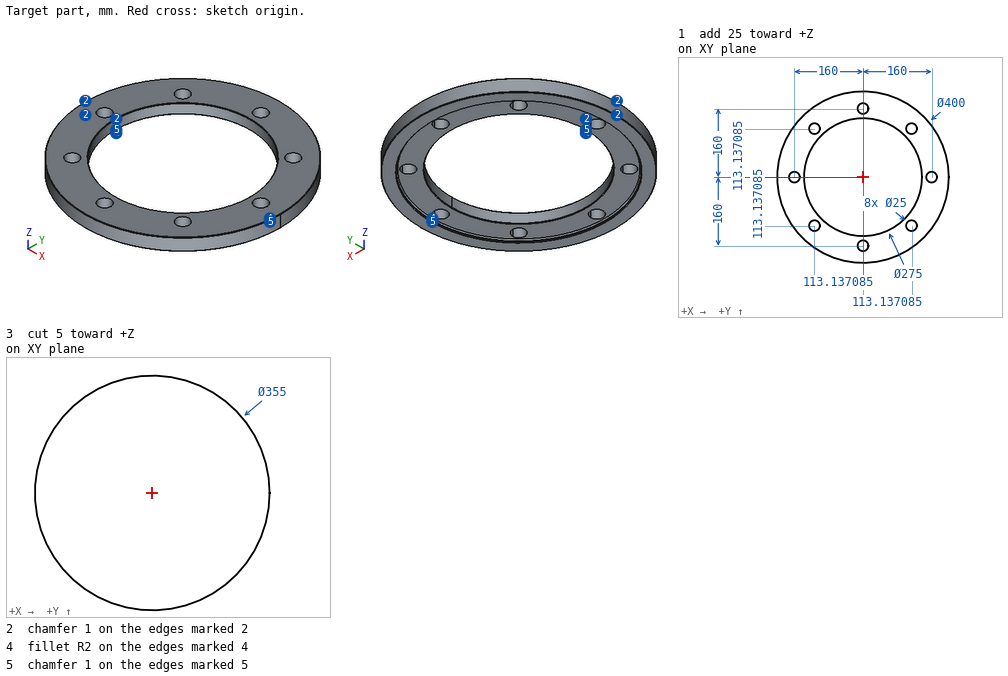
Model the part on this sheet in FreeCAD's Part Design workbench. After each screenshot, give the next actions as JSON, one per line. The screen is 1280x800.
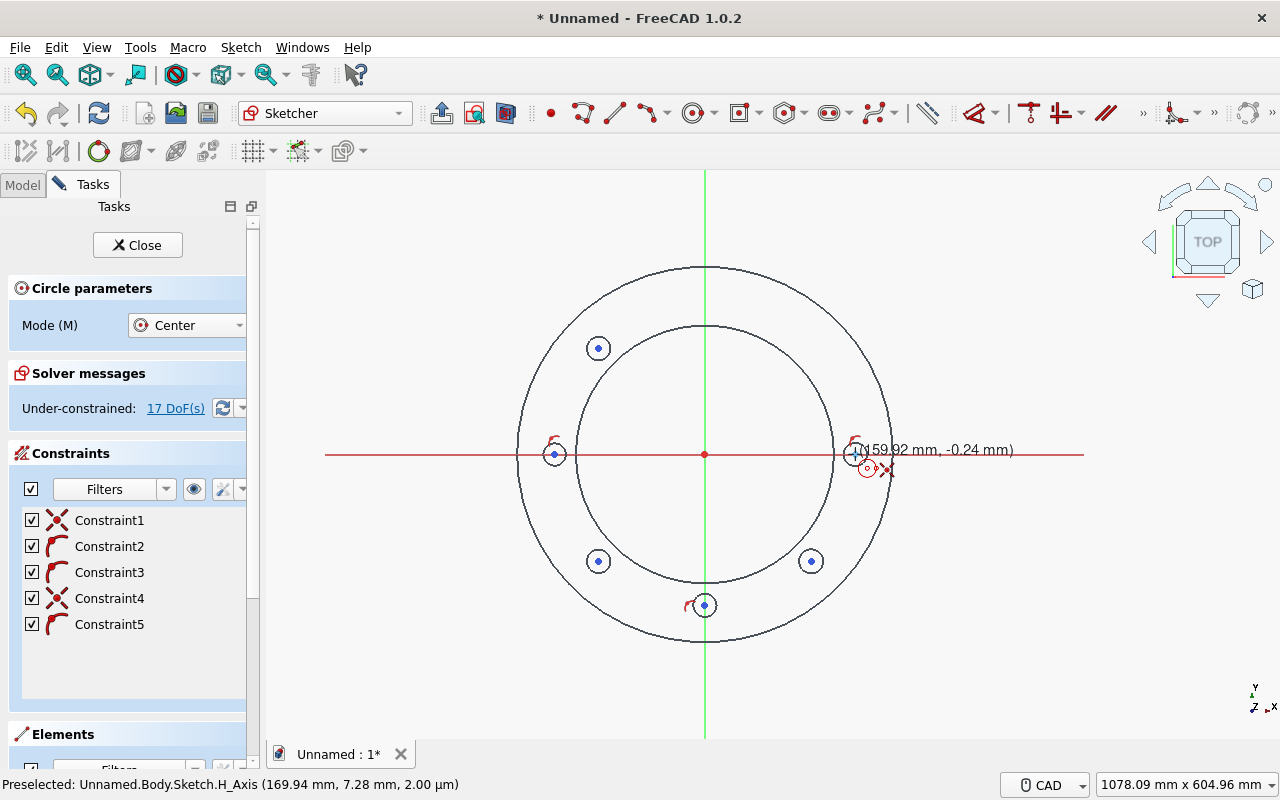
{"action": "scroll", "coordinate": [705, 304], "scroll_direction": "up", "scroll_amount": 4}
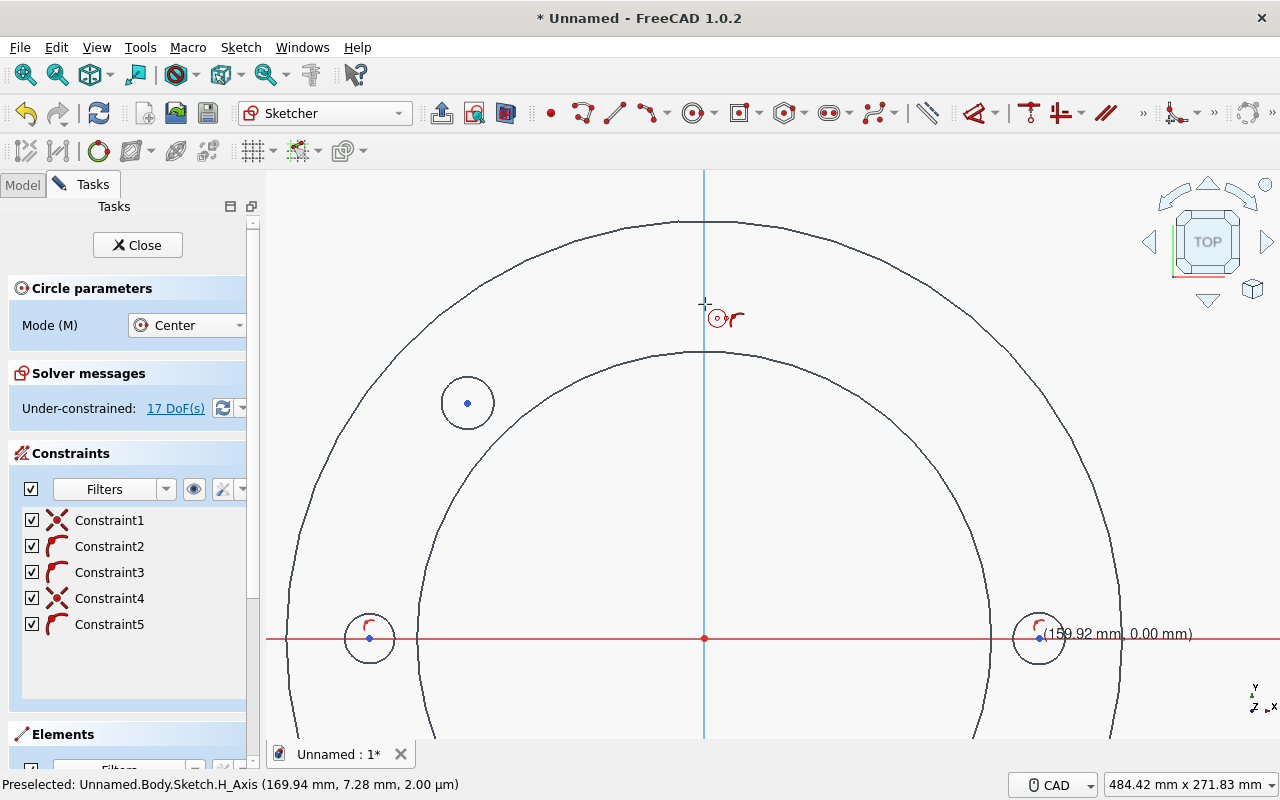
{"action": "left_click", "coordinate": [704, 304]}
{"action": "left_click", "coordinate": [723, 285]}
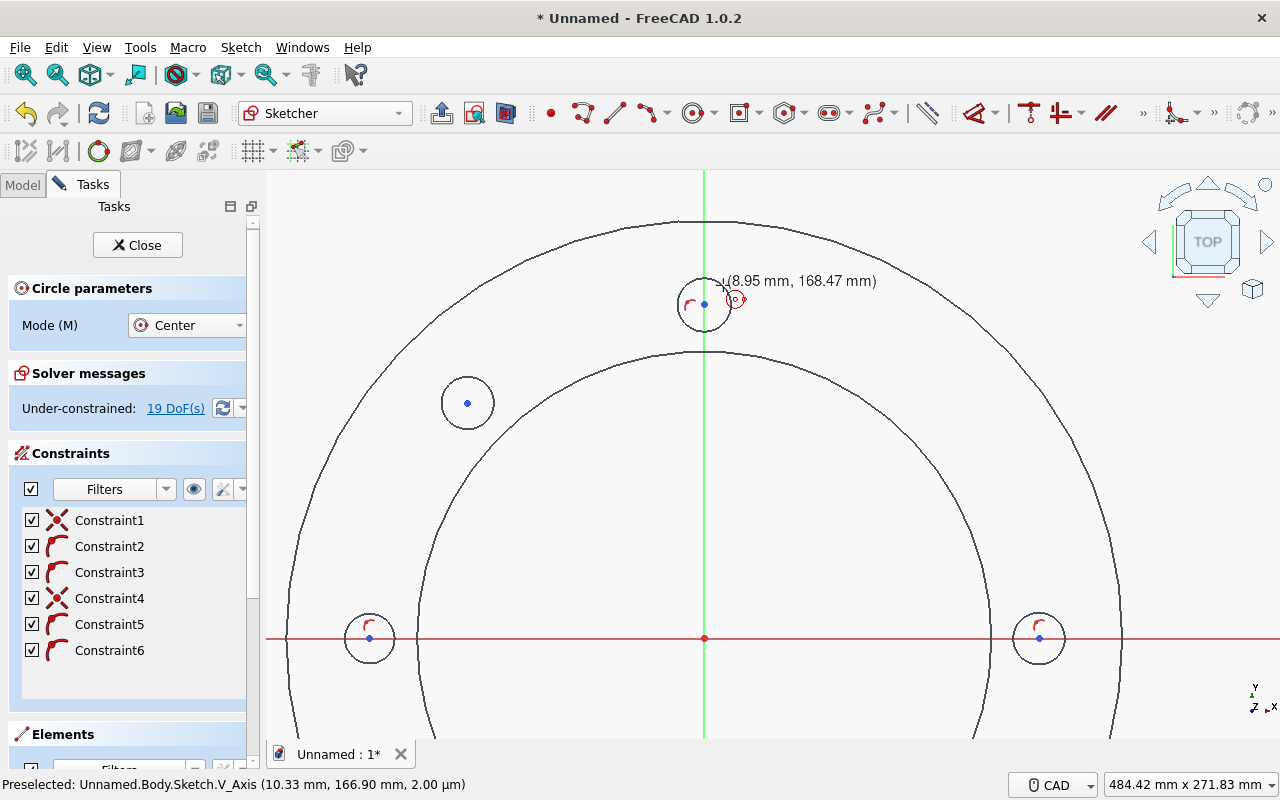
{"action": "left_click", "coordinate": [941, 402]}
{"action": "left_click", "coordinate": [960, 383]}
{"action": "key", "text": "Escape"}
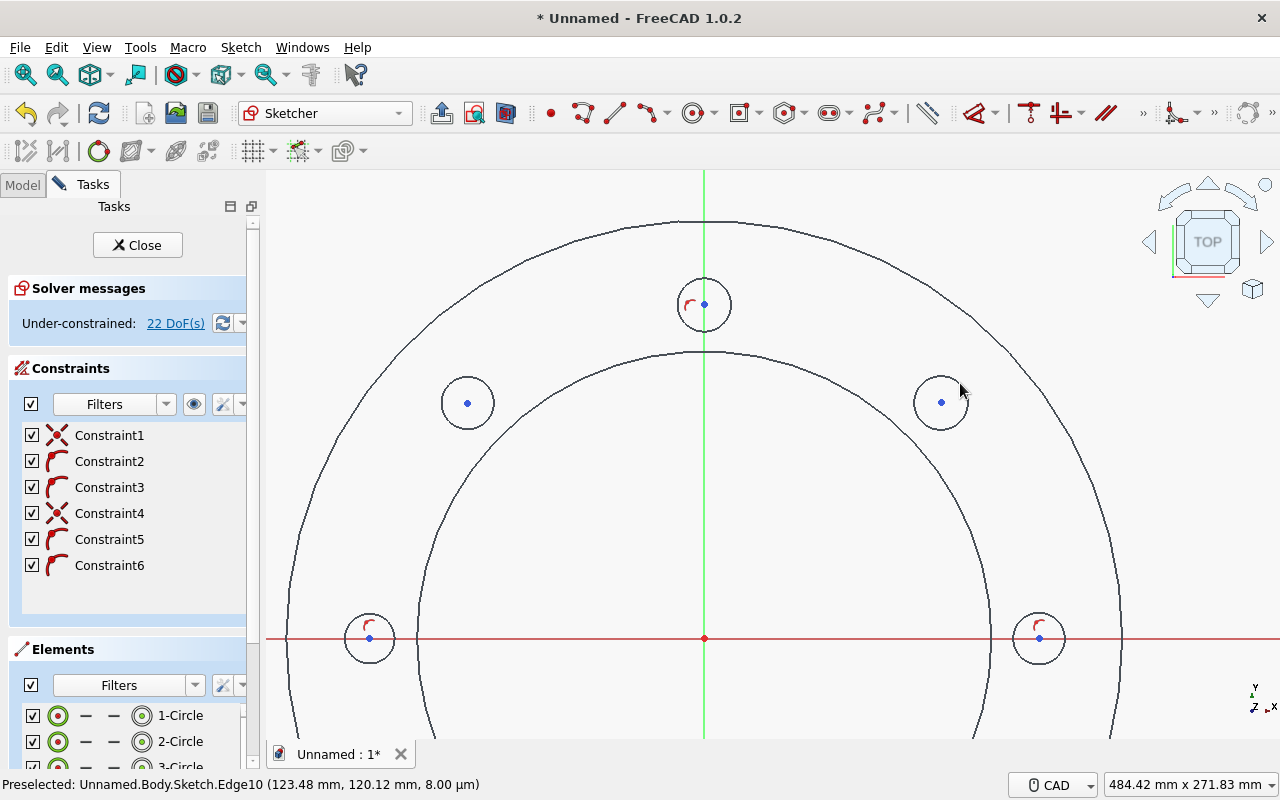
{"action": "scroll", "coordinate": [705, 304], "scroll_direction": "down", "scroll_amount": 4}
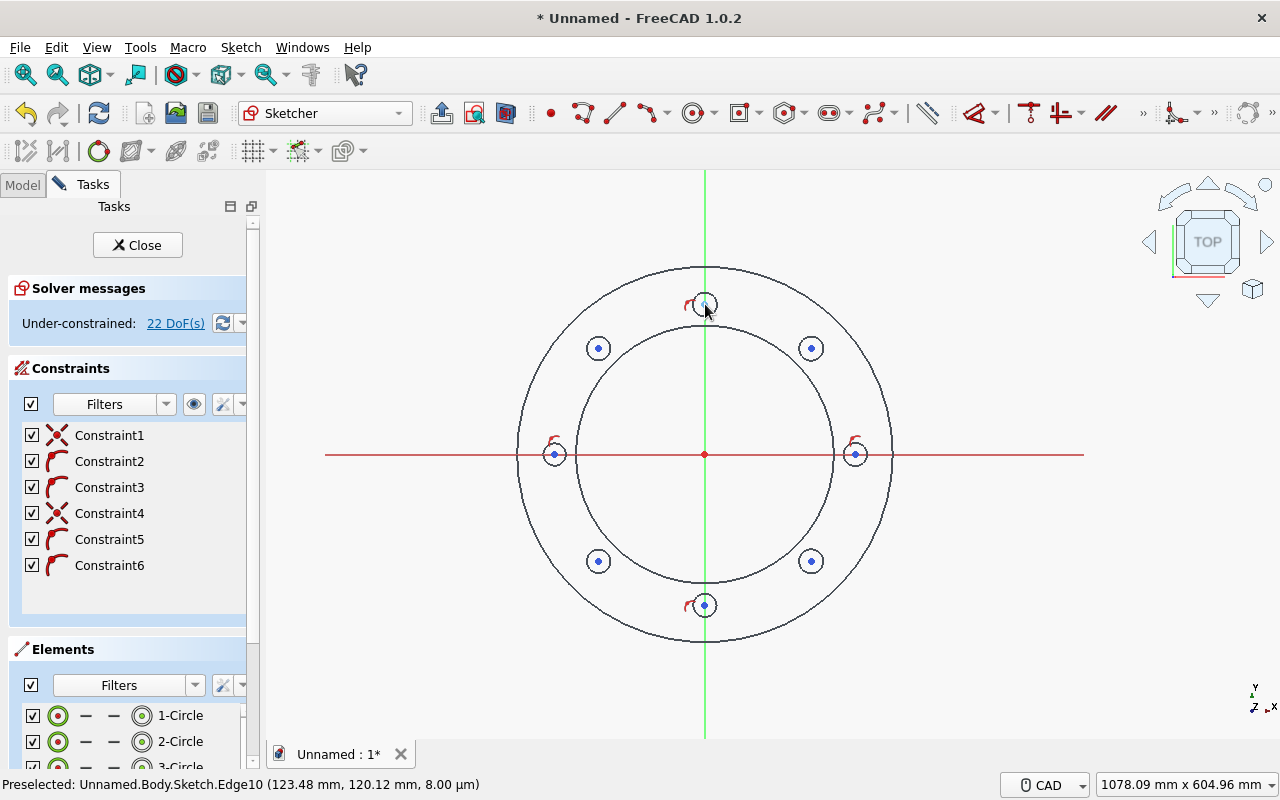
{"action": "scroll", "coordinate": [607, 553], "scroll_direction": "up", "scroll_amount": 2}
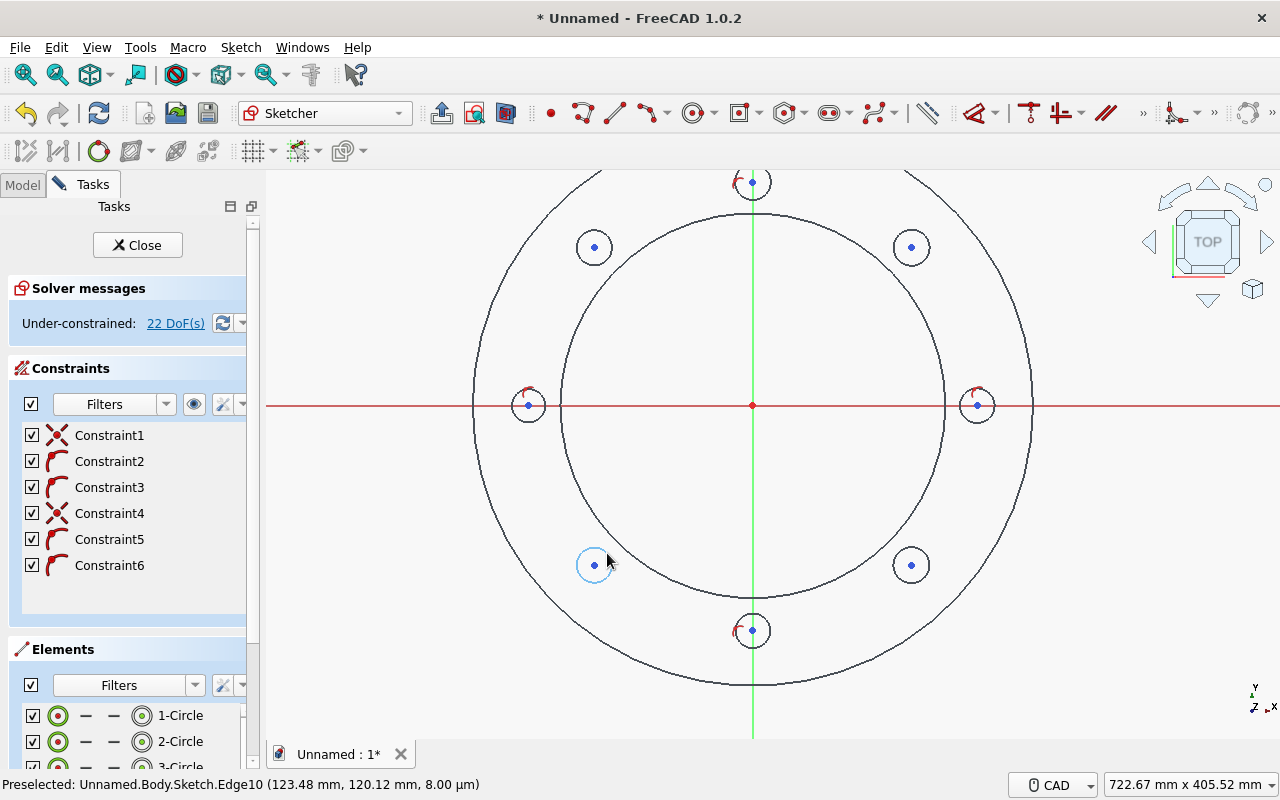
{"action": "left_click", "coordinate": [607, 553]}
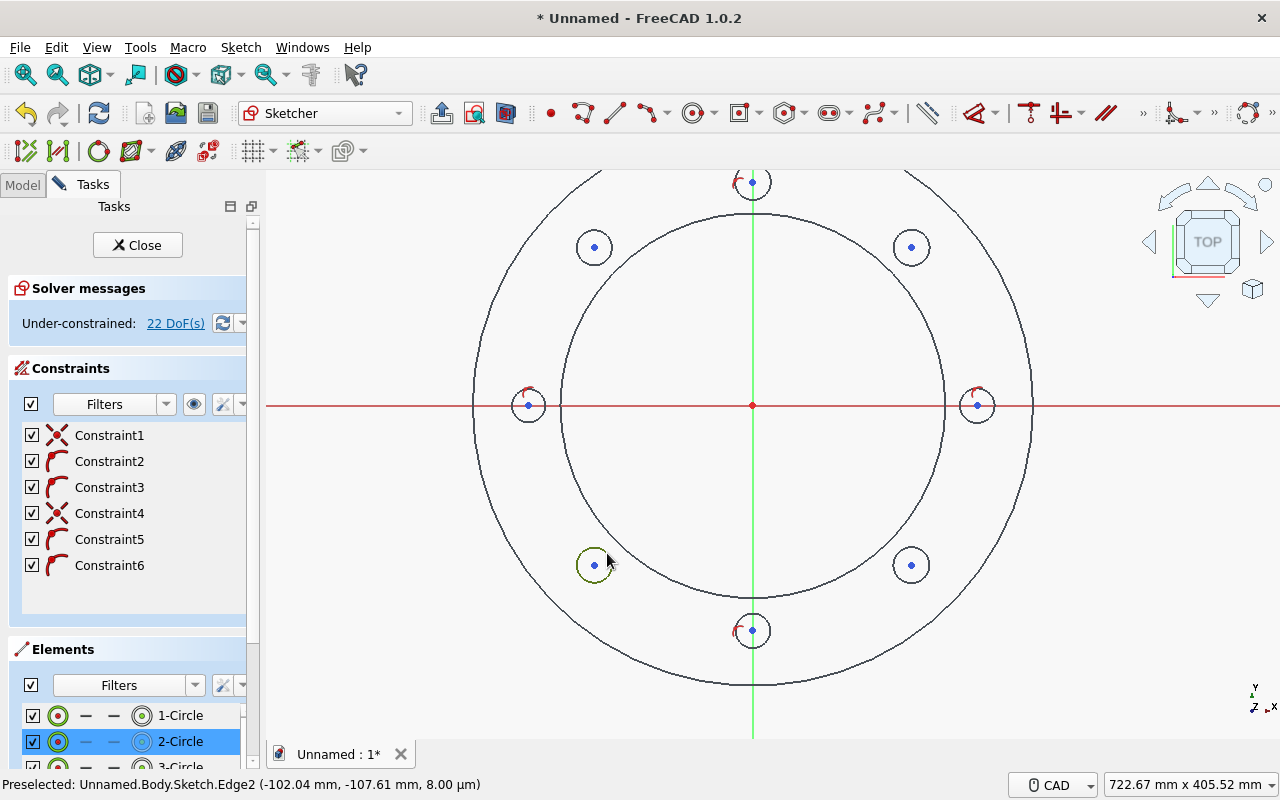
{"action": "left_click", "coordinate": [765, 619]}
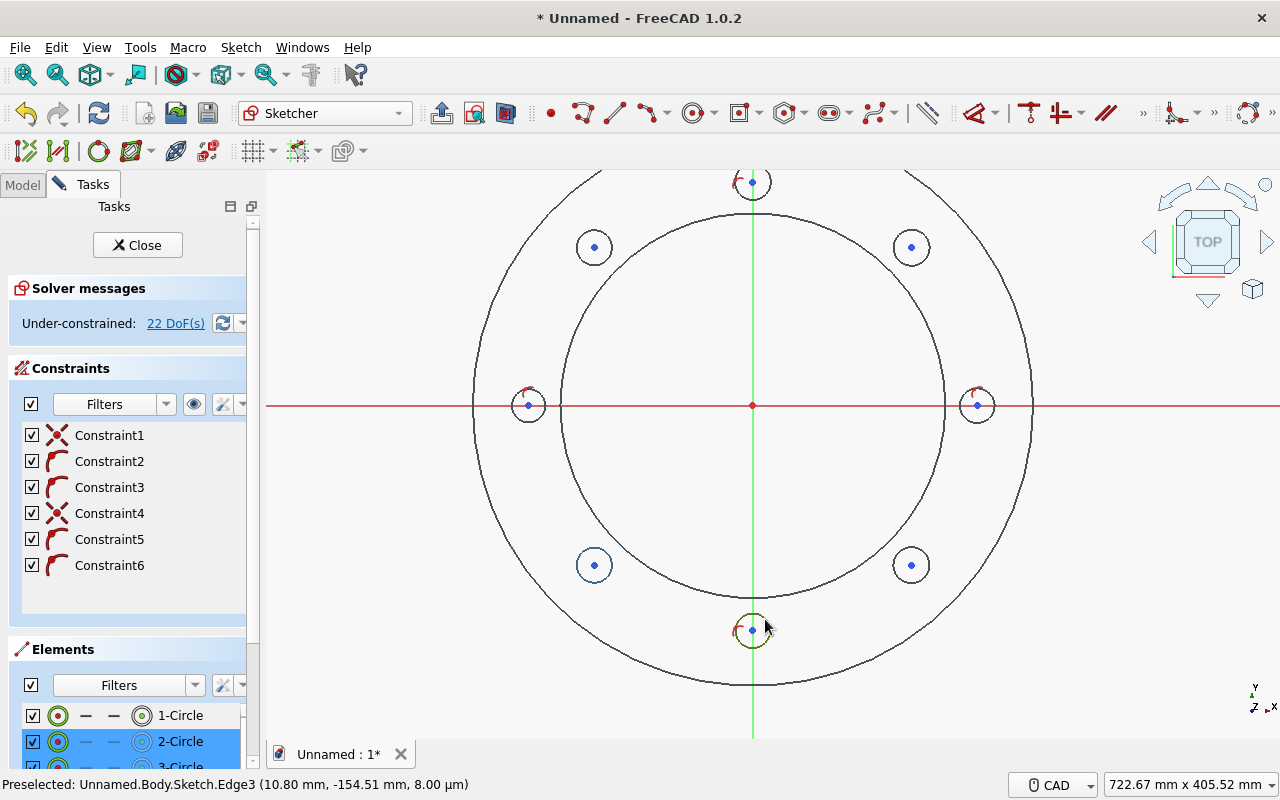
{"action": "left_click", "coordinate": [924, 552]}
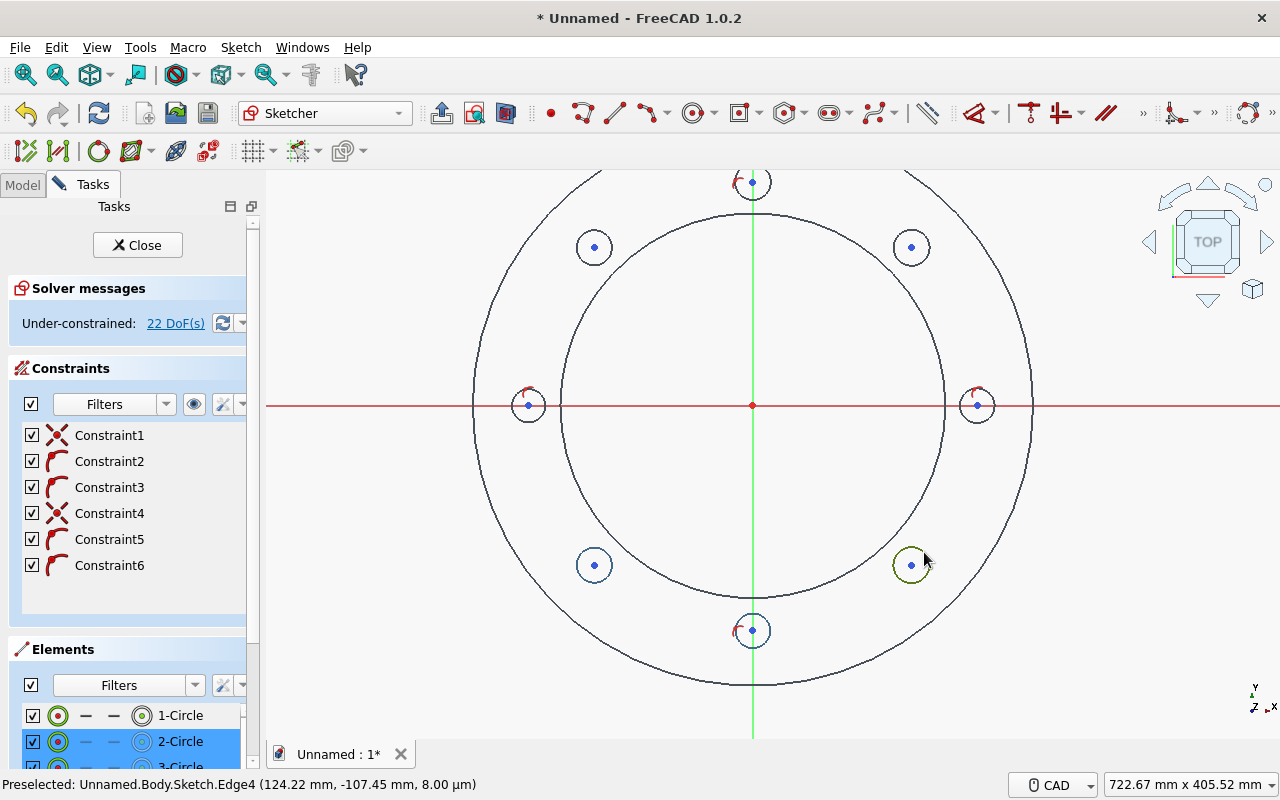
{"action": "left_click", "coordinate": [540, 394]}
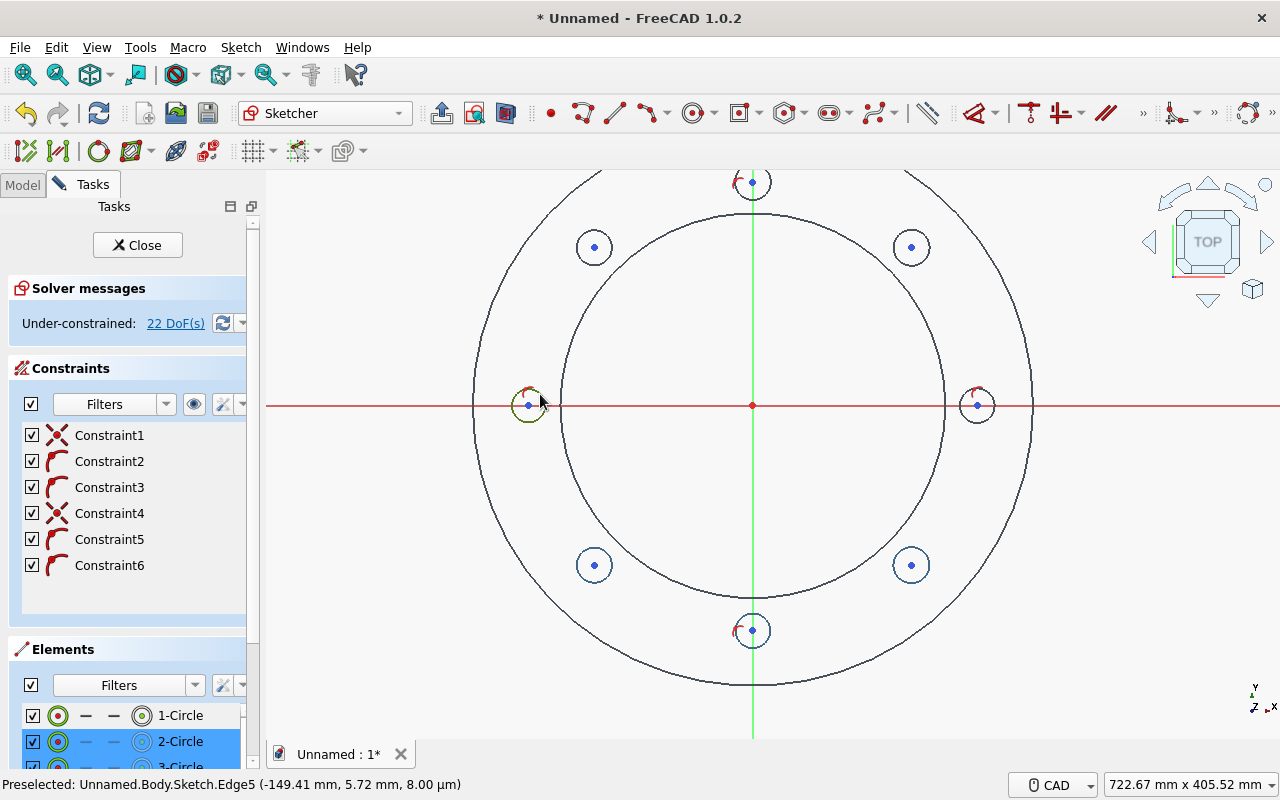
{"action": "left_click", "coordinate": [607, 235]}